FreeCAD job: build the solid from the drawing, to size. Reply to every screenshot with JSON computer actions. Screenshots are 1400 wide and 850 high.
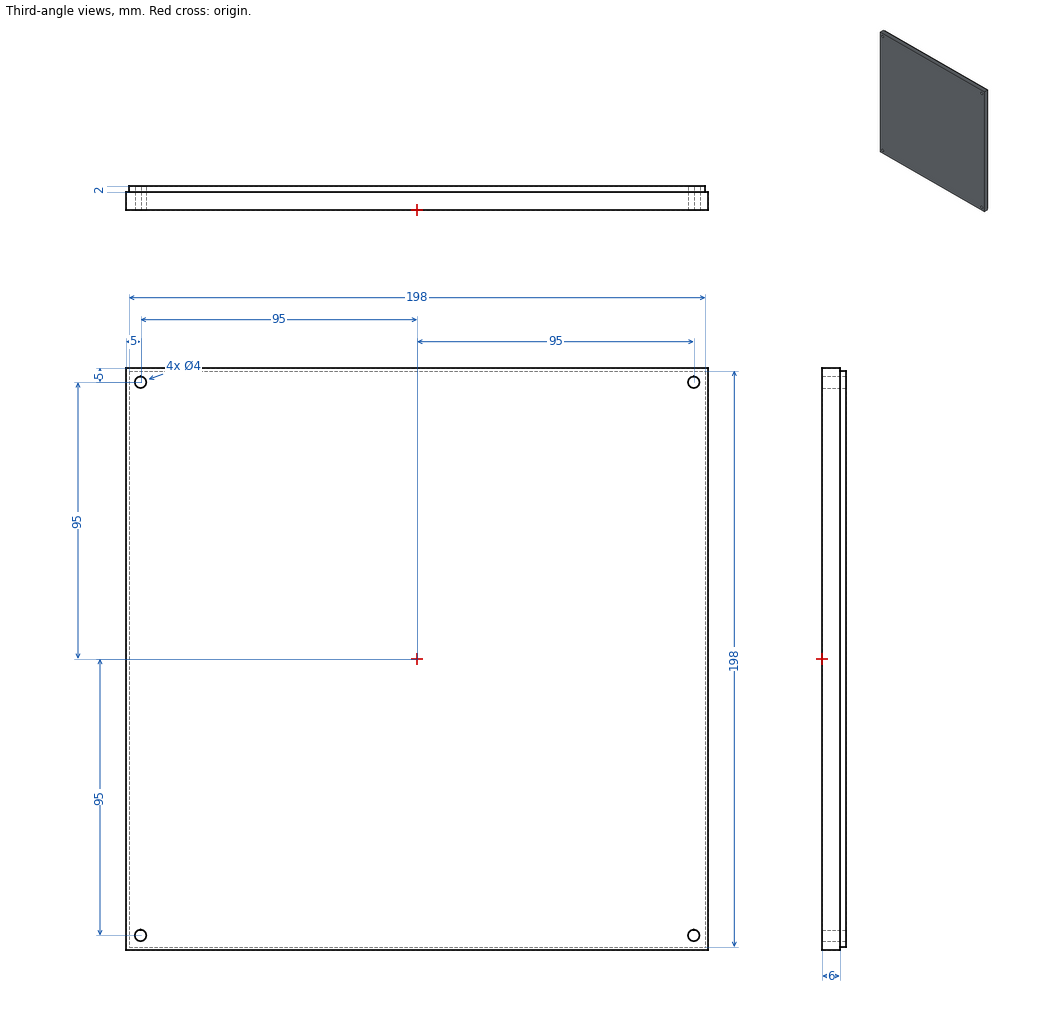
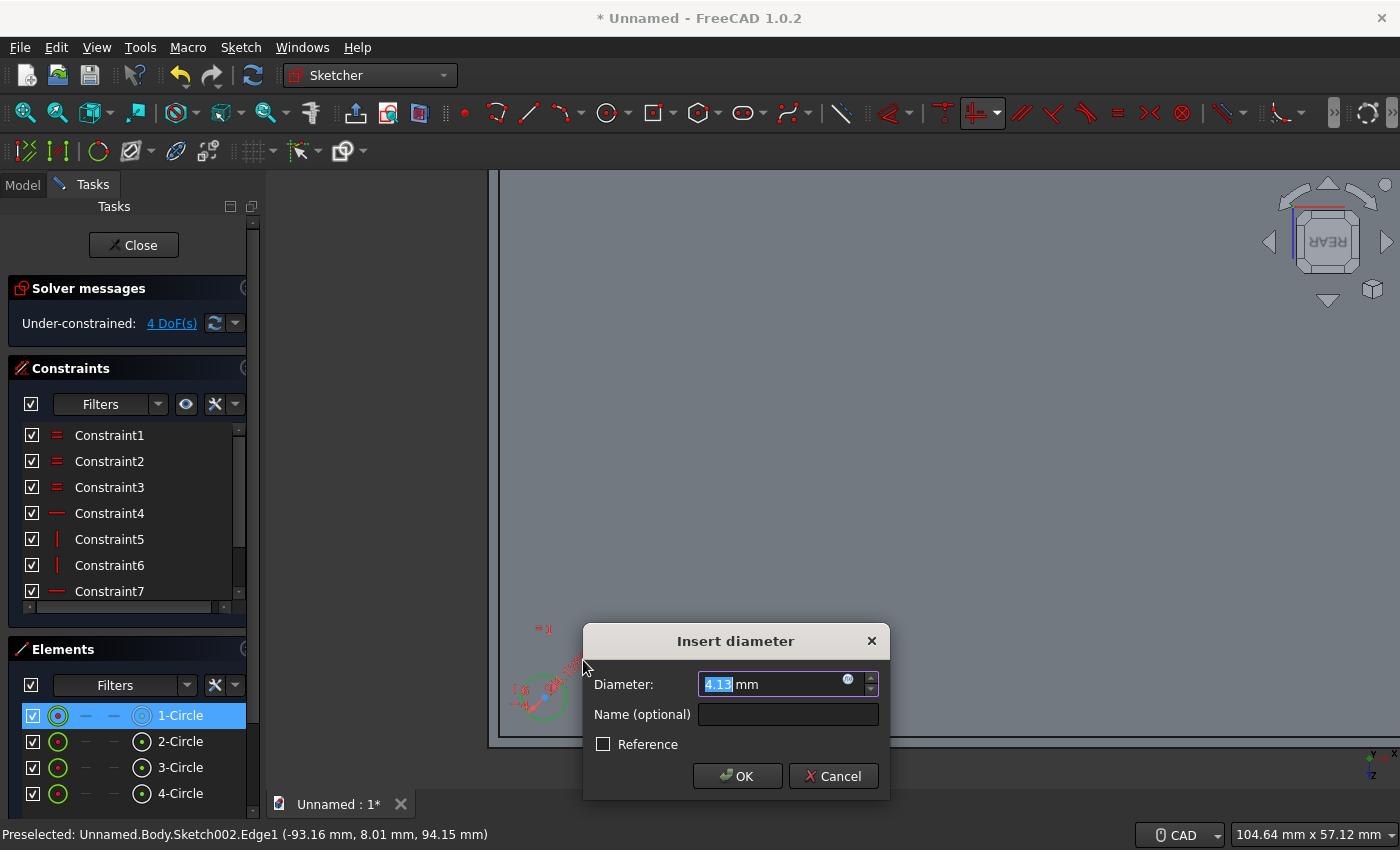
{"action": "type", "text": "4"}
{"action": "key", "text": "Return"}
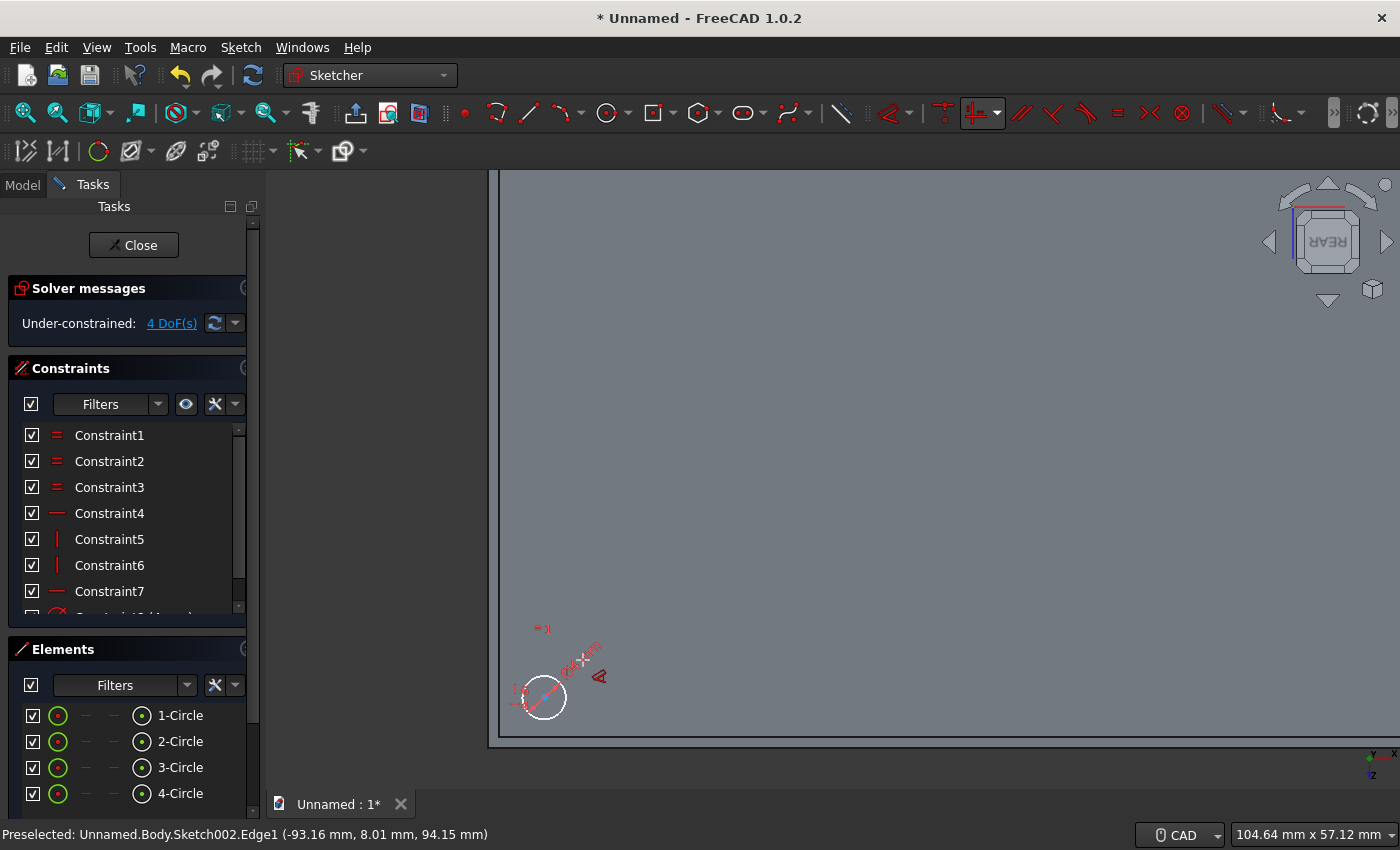
{"action": "scroll", "coordinate": [560, 686], "scroll_direction": "down", "scroll_amount": 8}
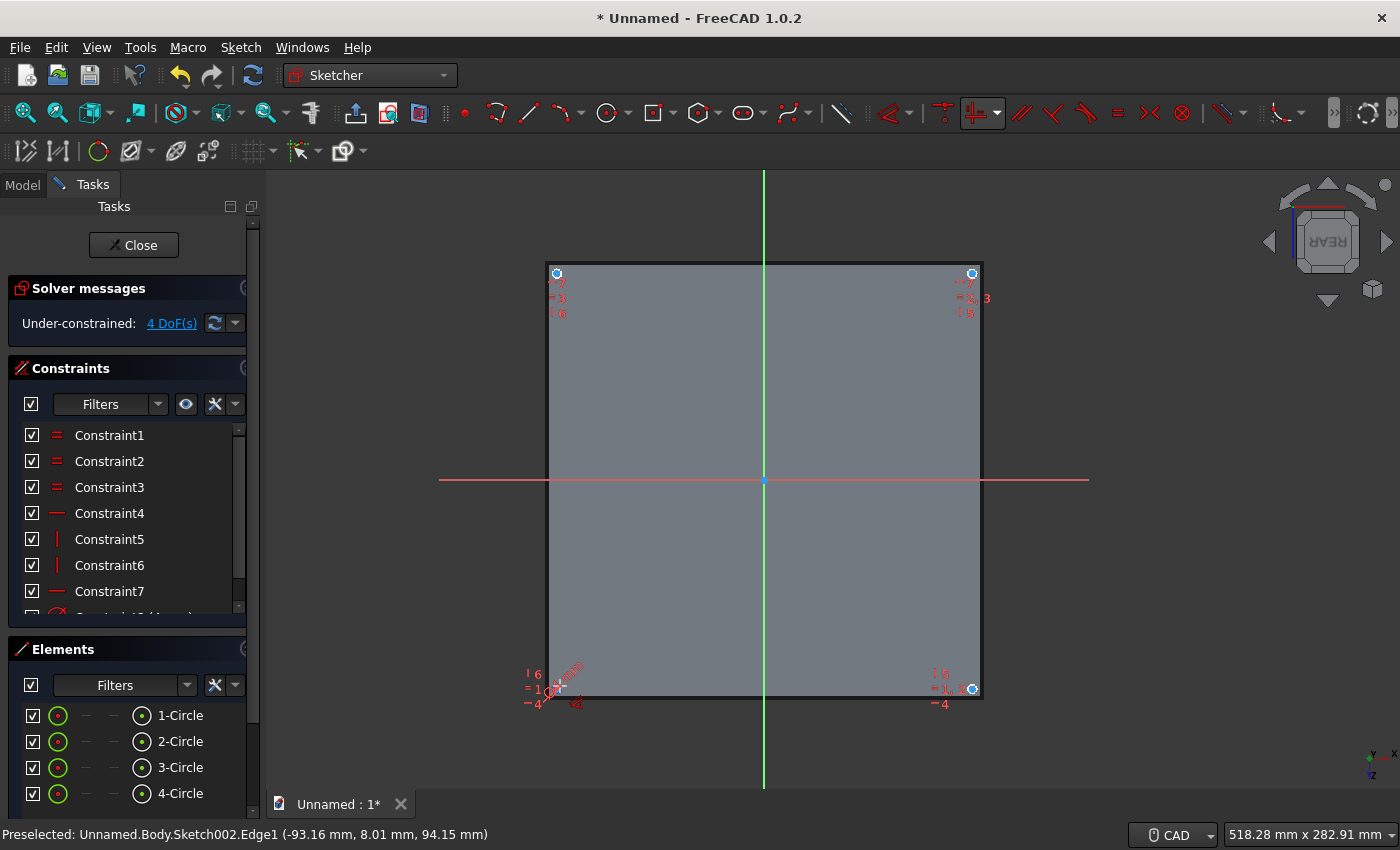
{"action": "left_click", "coordinate": [557, 689]}
{"action": "left_click", "coordinate": [661, 723]}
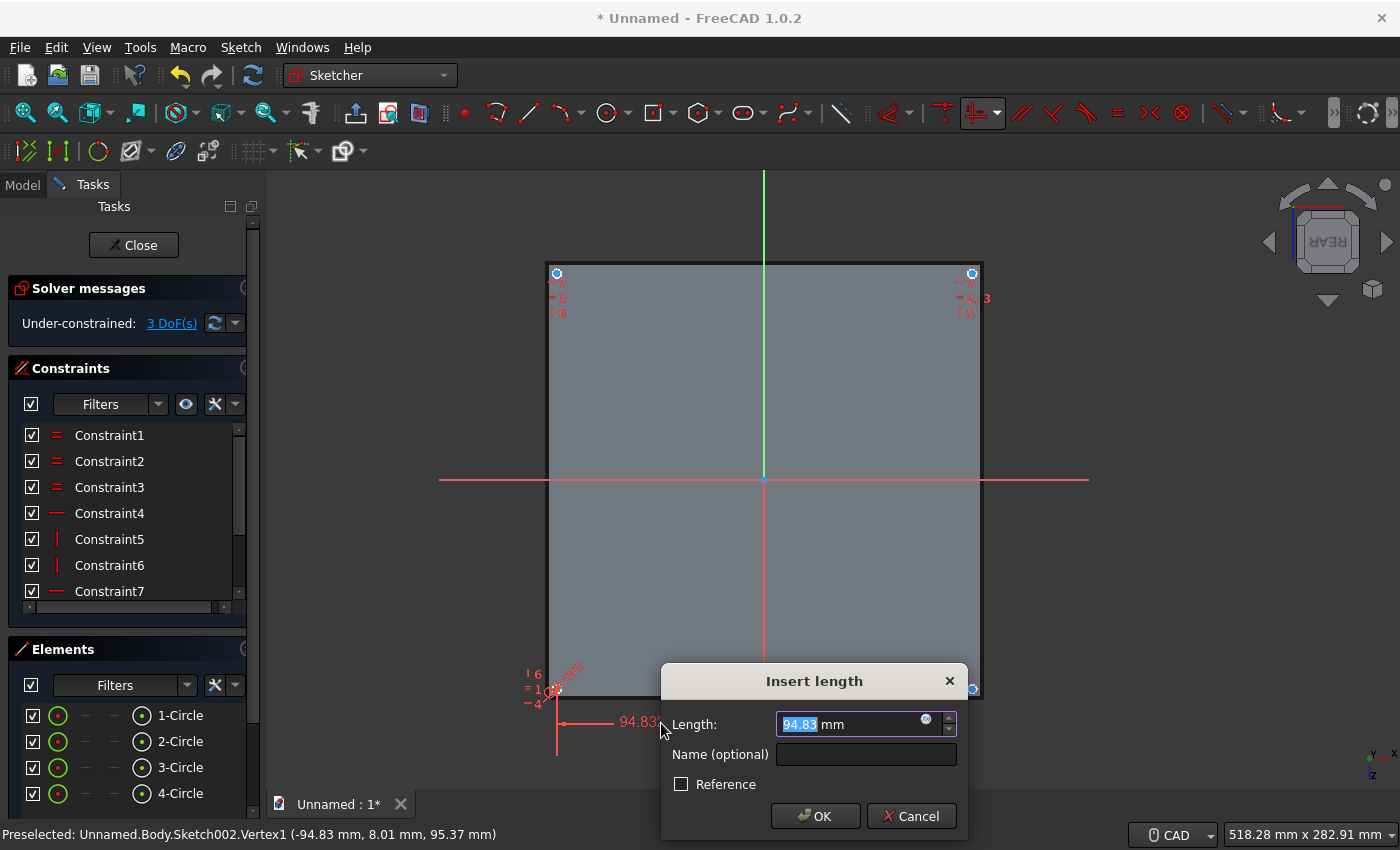
{"action": "type", "text": "95"}
{"action": "key", "text": "Return"}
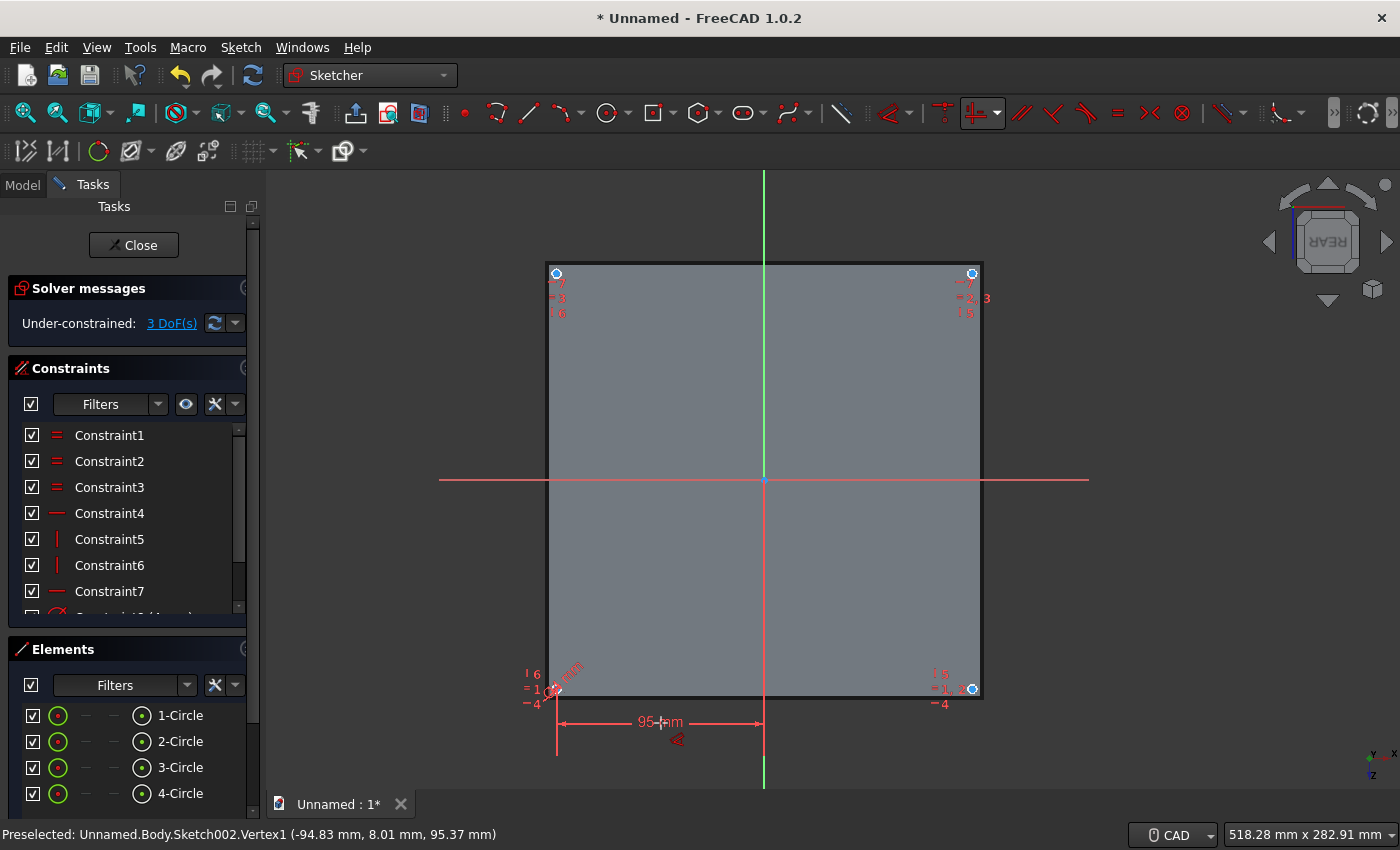
{"action": "left_click", "coordinate": [557, 689]}
{"action": "left_click", "coordinate": [523, 585]}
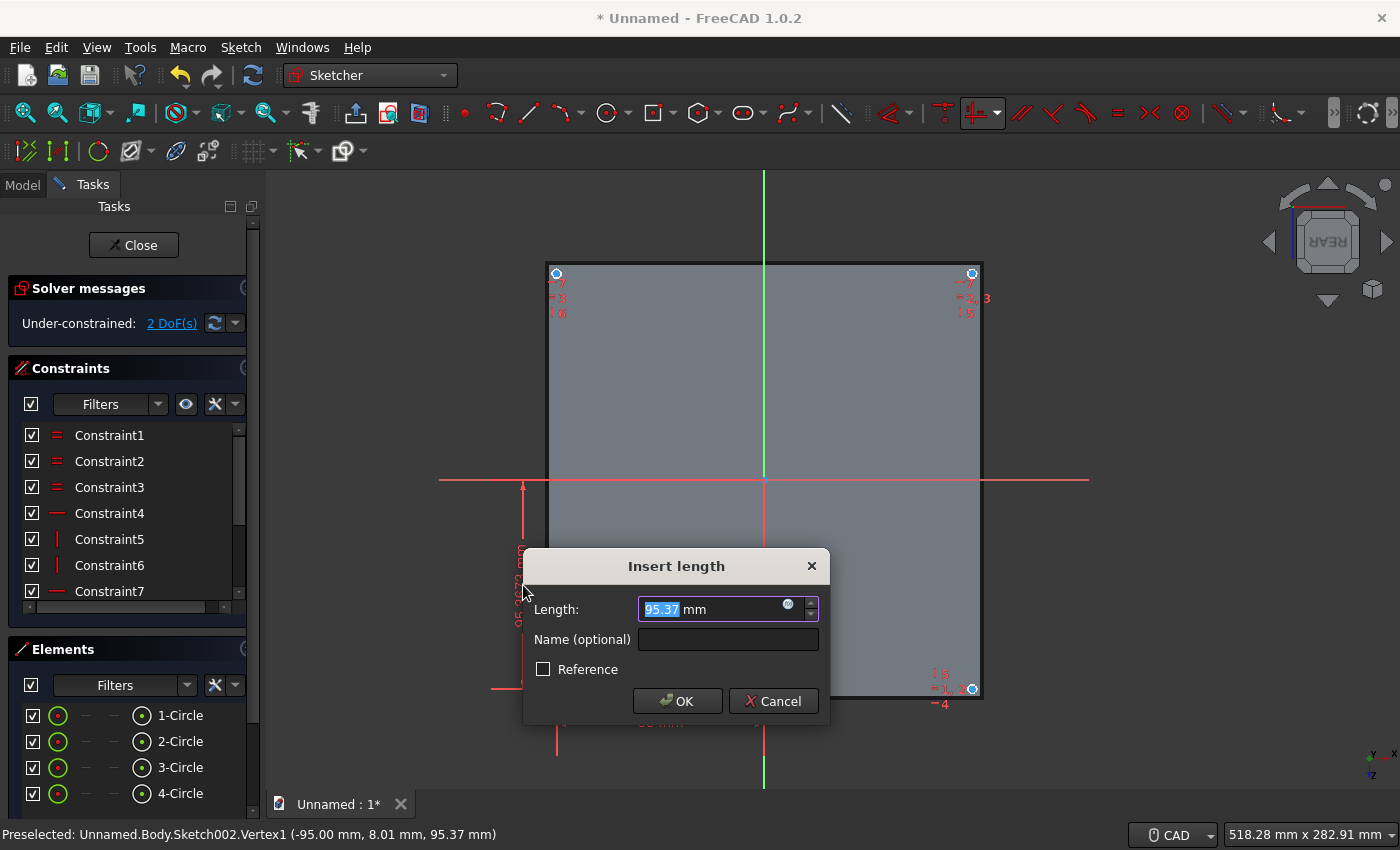
{"action": "type", "text": "95"}
{"action": "key", "text": "Return"}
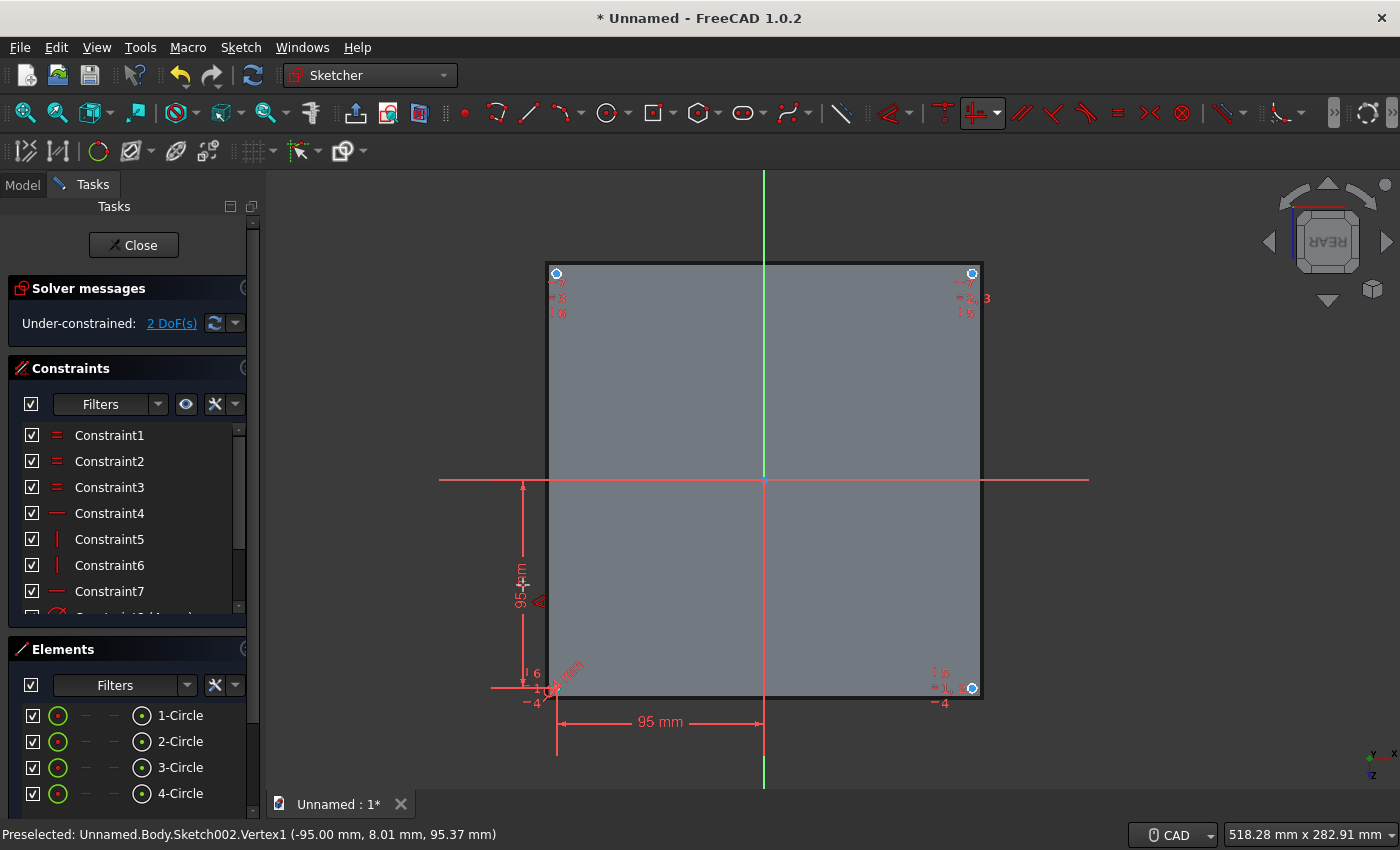
{"action": "left_click", "coordinate": [972, 688]}
{"action": "left_click", "coordinate": [868, 722]}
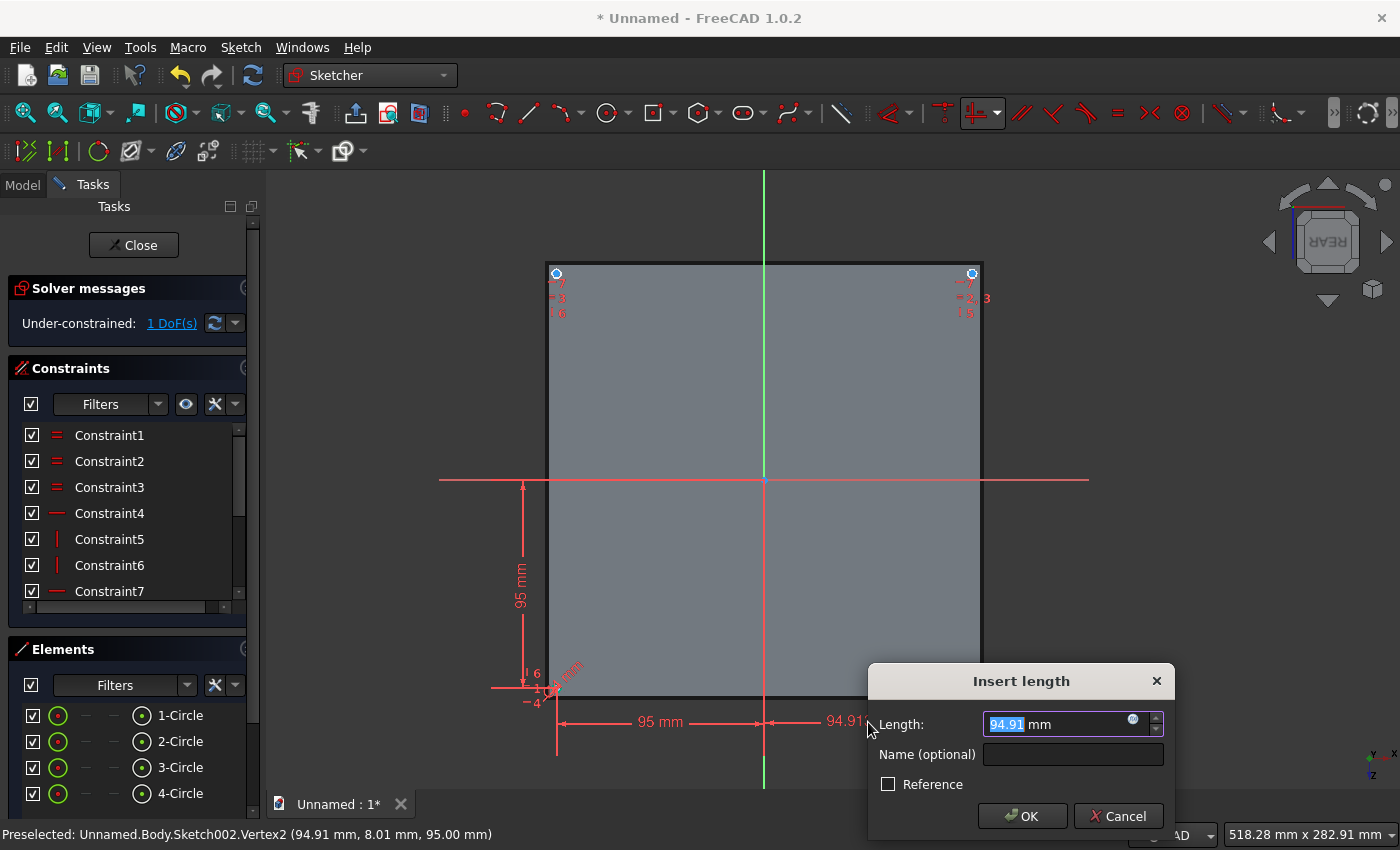
{"action": "type", "text": "95"}
{"action": "key", "text": "Return"}